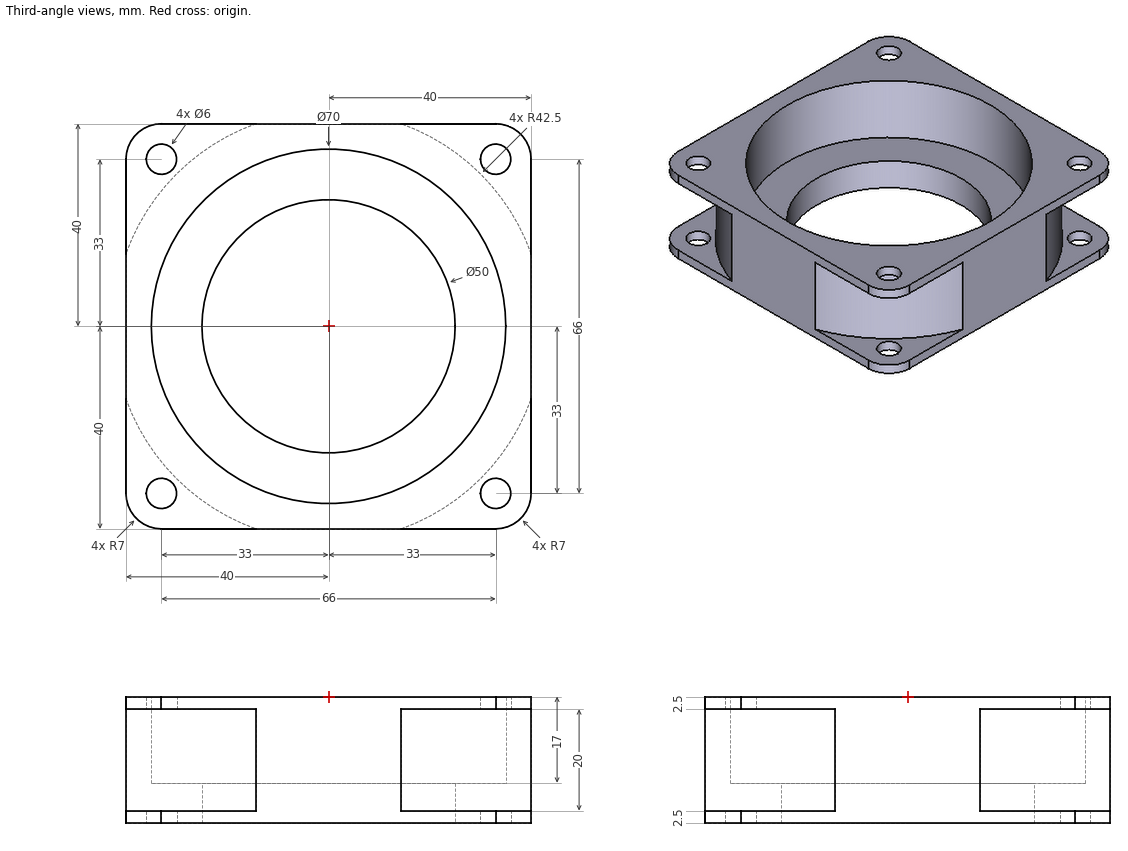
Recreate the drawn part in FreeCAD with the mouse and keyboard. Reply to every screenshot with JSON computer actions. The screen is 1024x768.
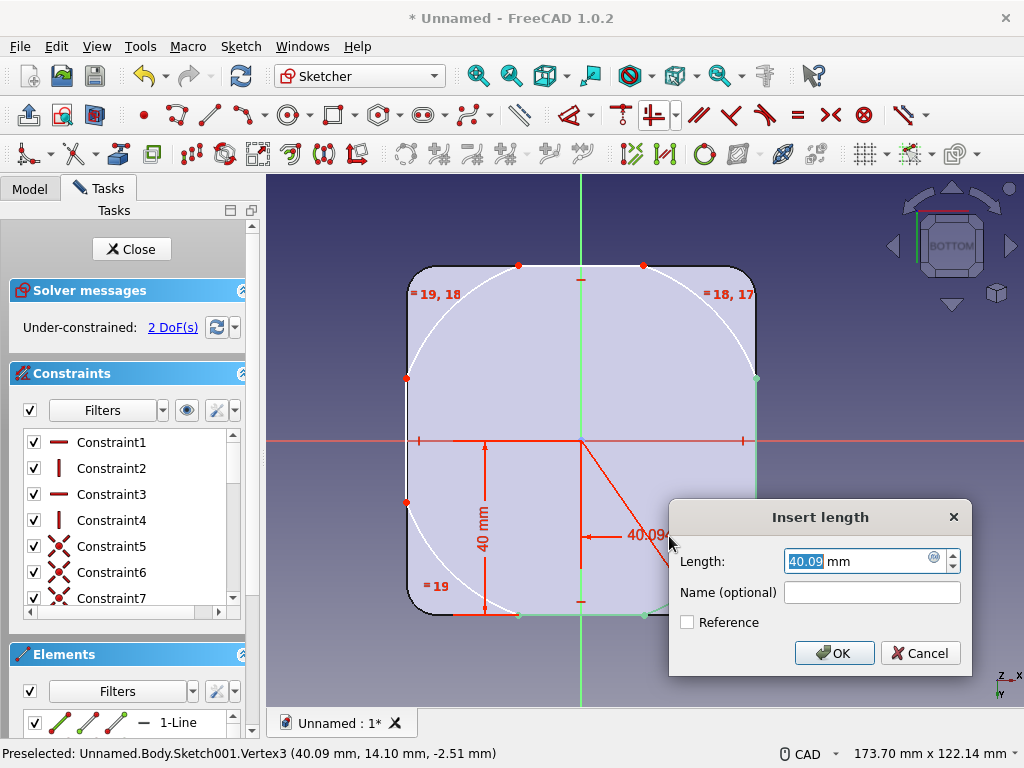
{"action": "type", "text": "40"}
{"action": "key", "text": "Return"}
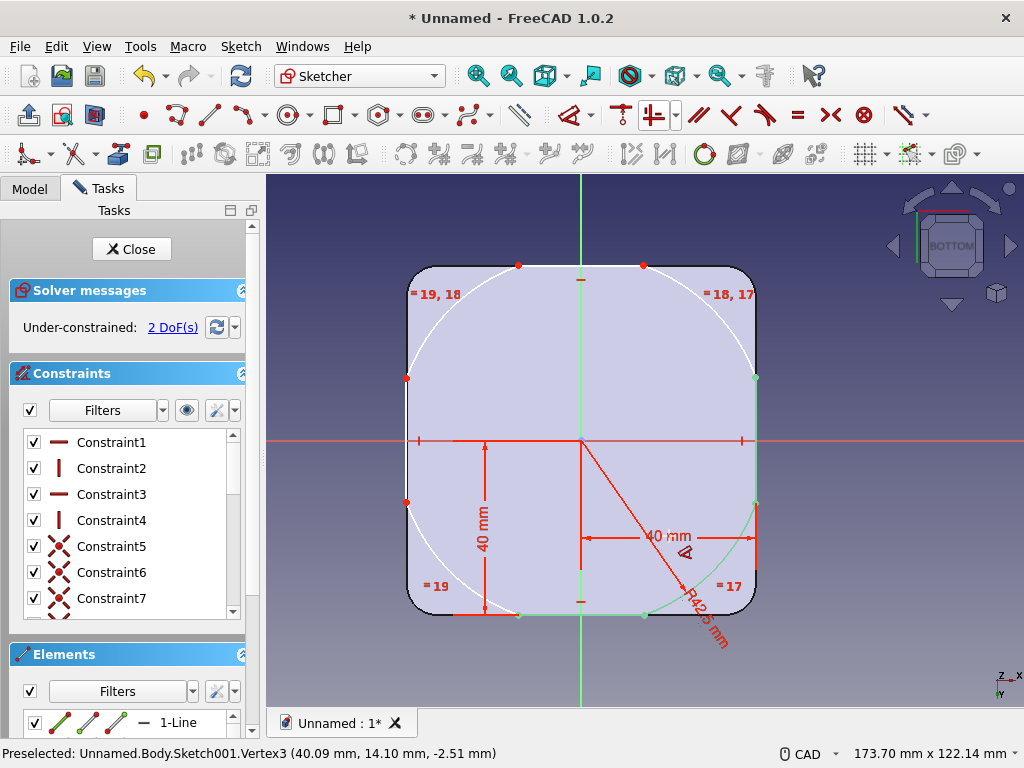
{"action": "left_click", "coordinate": [644, 266]}
{"action": "left_click", "coordinate": [678, 353]}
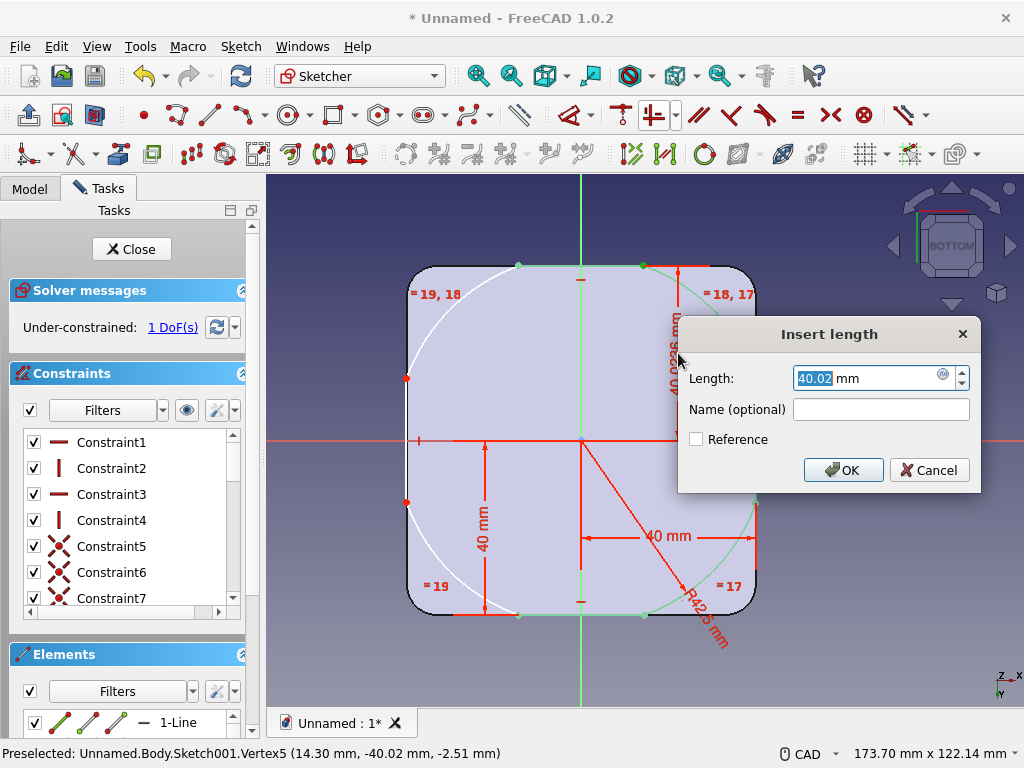
{"action": "type", "text": "40"}
{"action": "key", "text": "Return"}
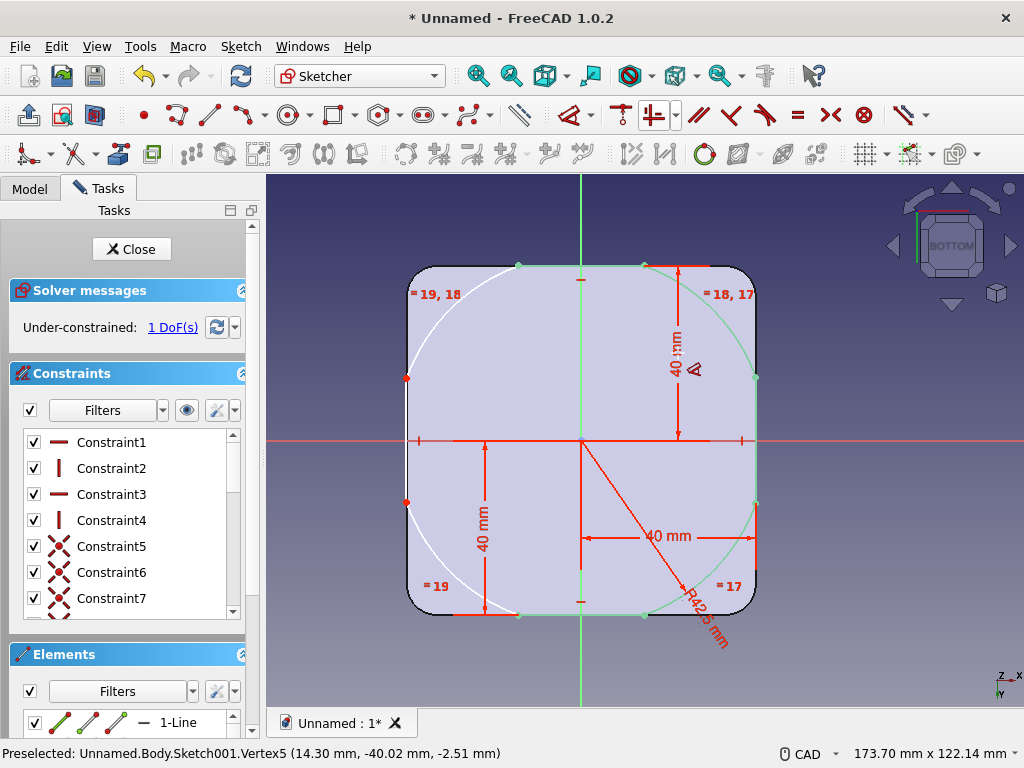
{"action": "left_click", "coordinate": [406, 379]}
{"action": "left_click", "coordinate": [494, 345]}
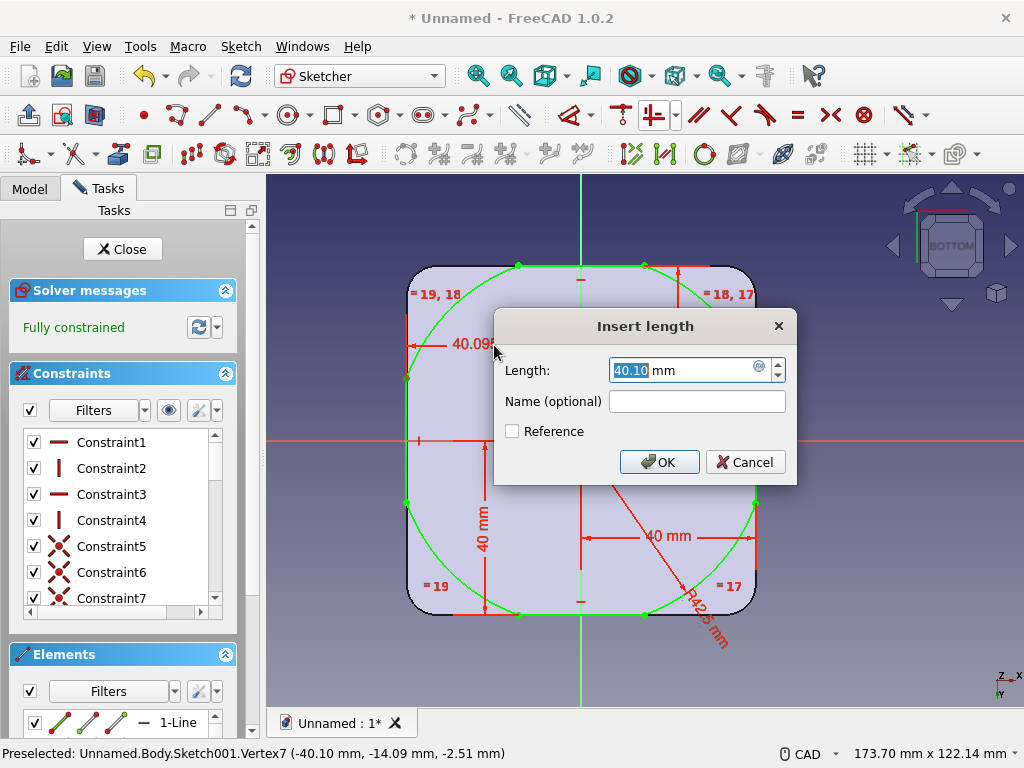
{"action": "type", "text": "40"}
{"action": "key", "text": "Return"}
{"action": "key", "text": "Escape"}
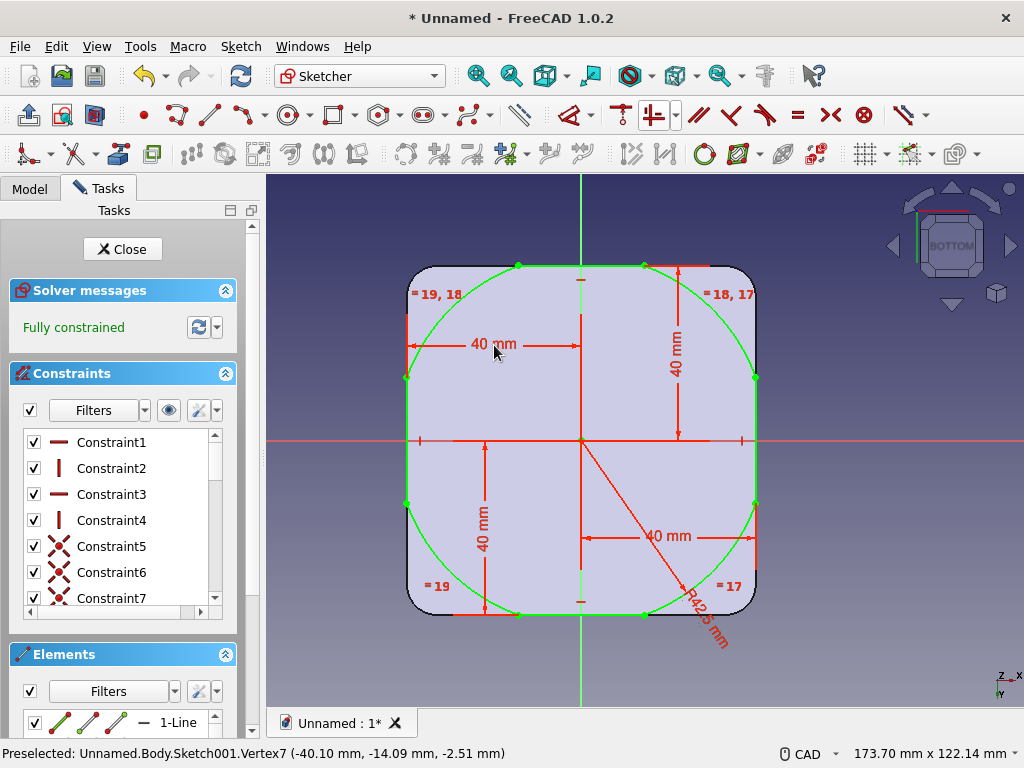
{"action": "left_click", "coordinate": [123, 249]}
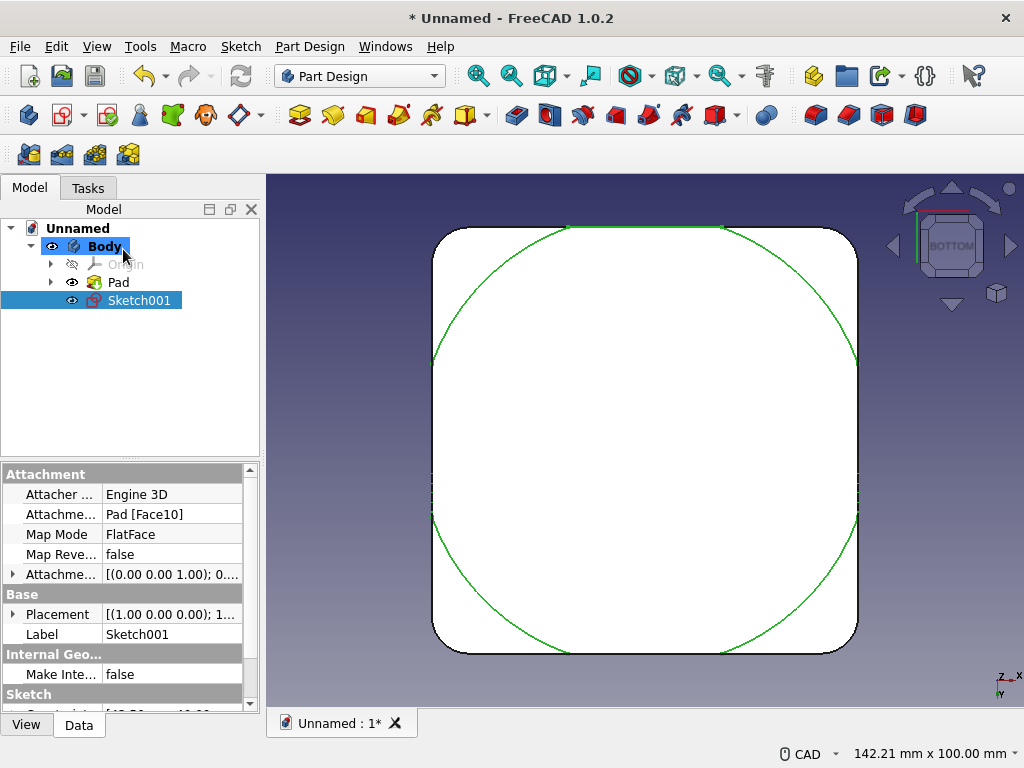
{"action": "left_click", "coordinate": [300, 116]}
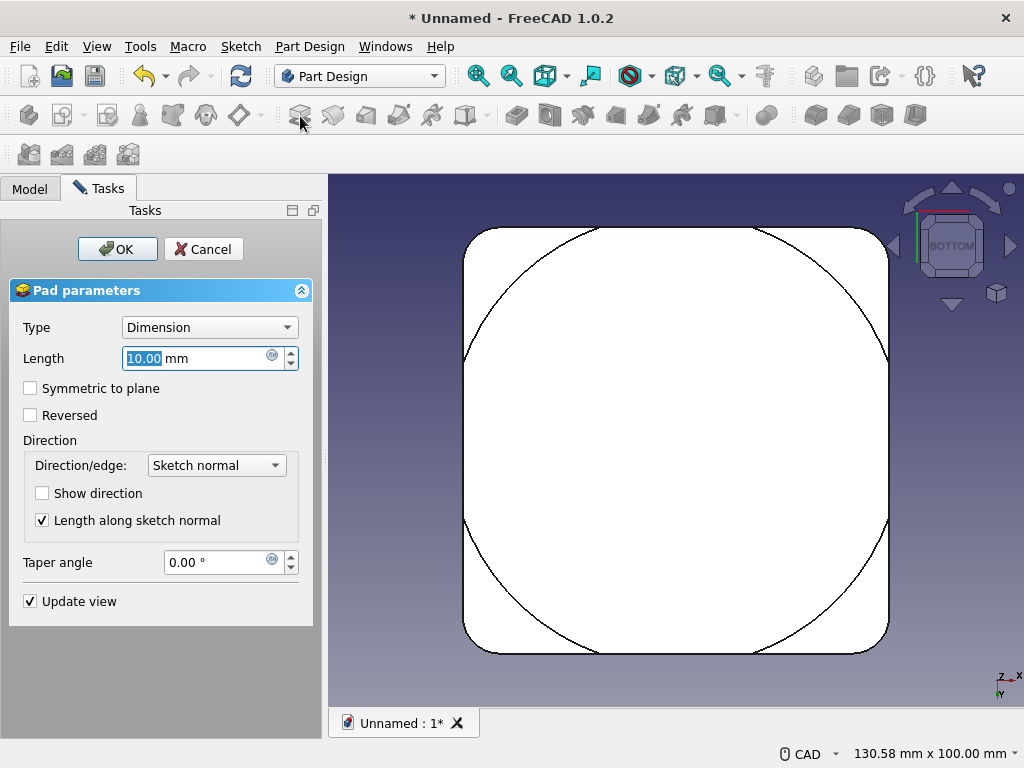
{"action": "type", "text": "20"}
{"action": "key", "text": "Tab"}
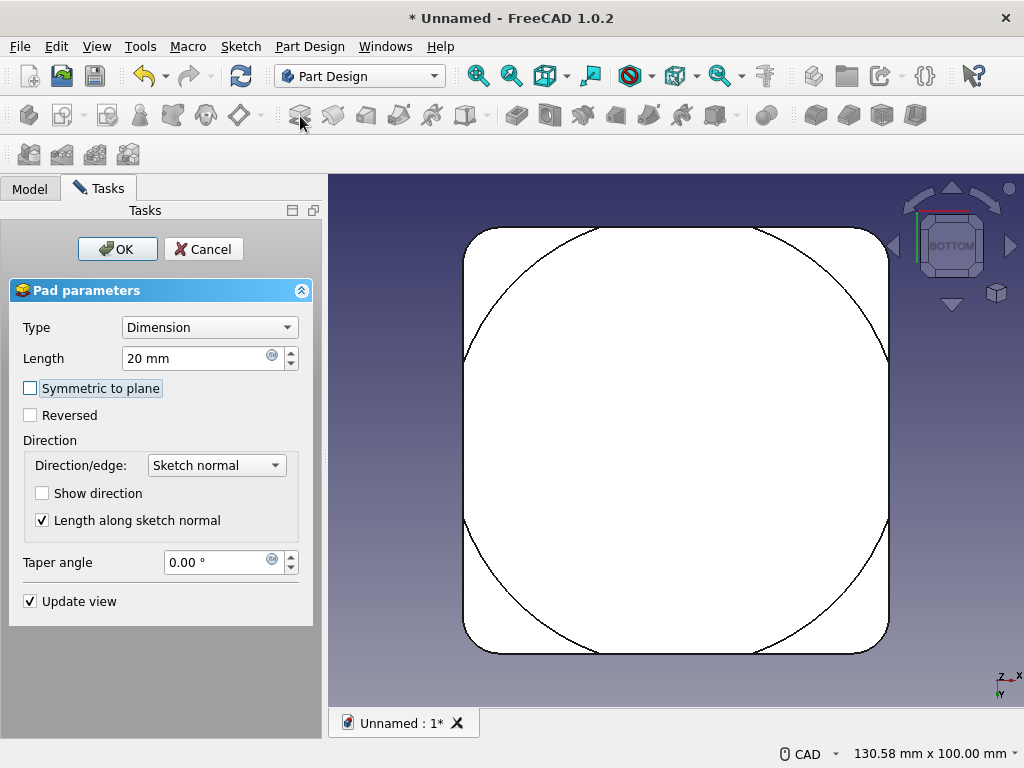
{"action": "left_click", "coordinate": [118, 249]}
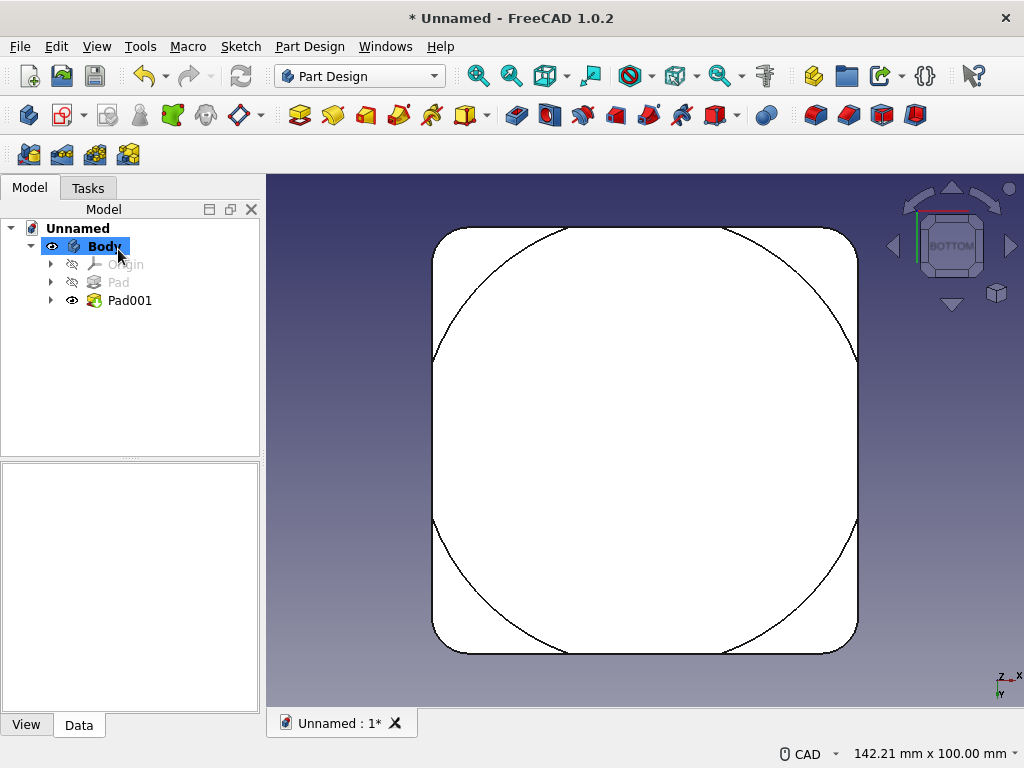
{"action": "left_click", "coordinate": [645, 440]}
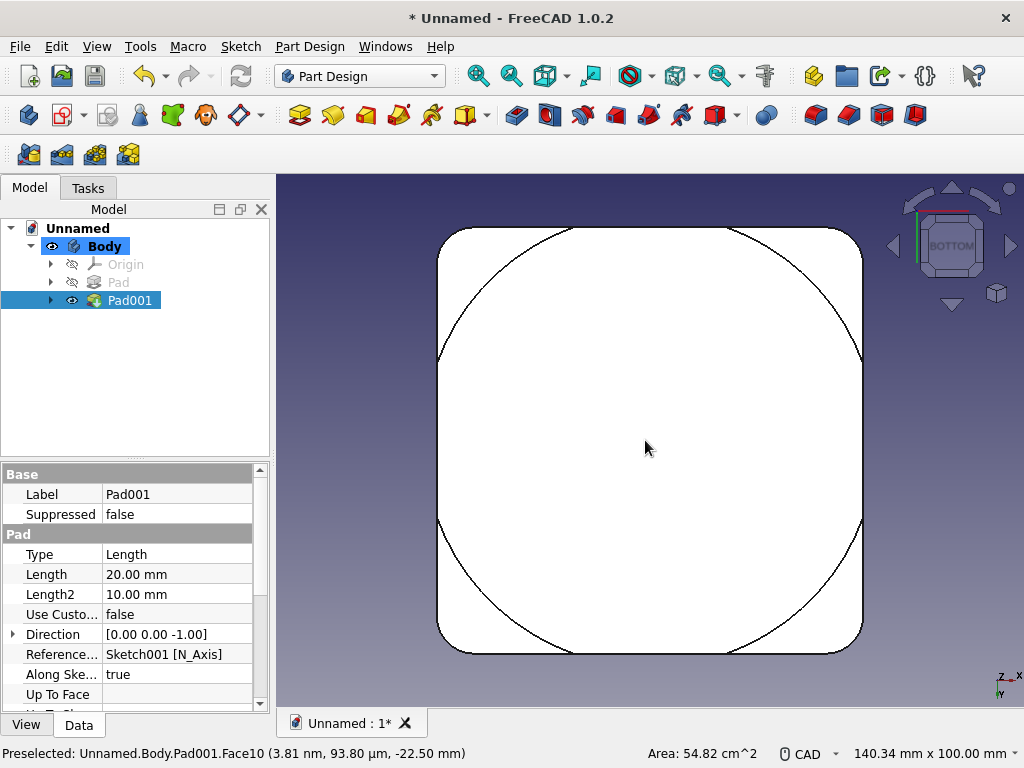
{"action": "left_click", "coordinate": [62, 116]}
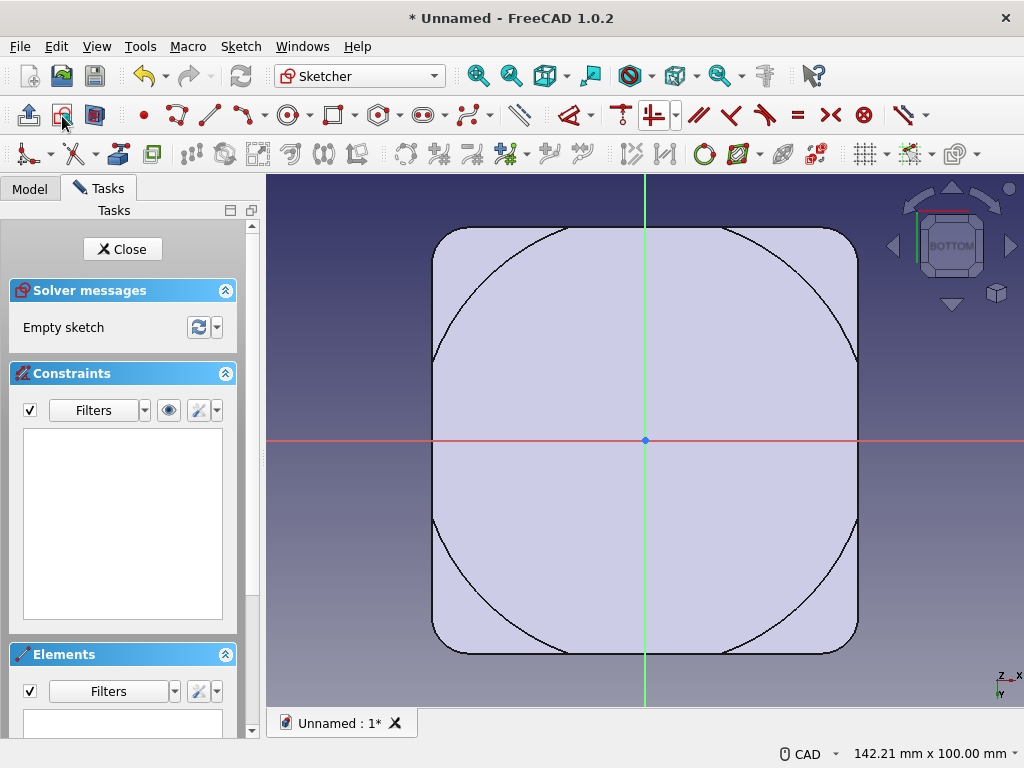
{"action": "scroll", "coordinate": [294, 440], "scroll_direction": "down", "scroll_amount": 1}